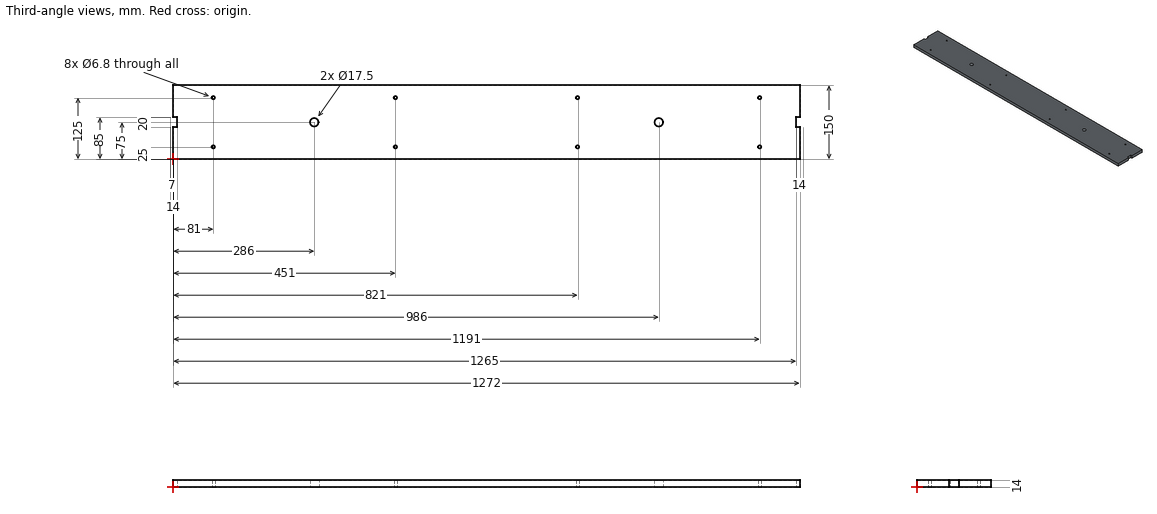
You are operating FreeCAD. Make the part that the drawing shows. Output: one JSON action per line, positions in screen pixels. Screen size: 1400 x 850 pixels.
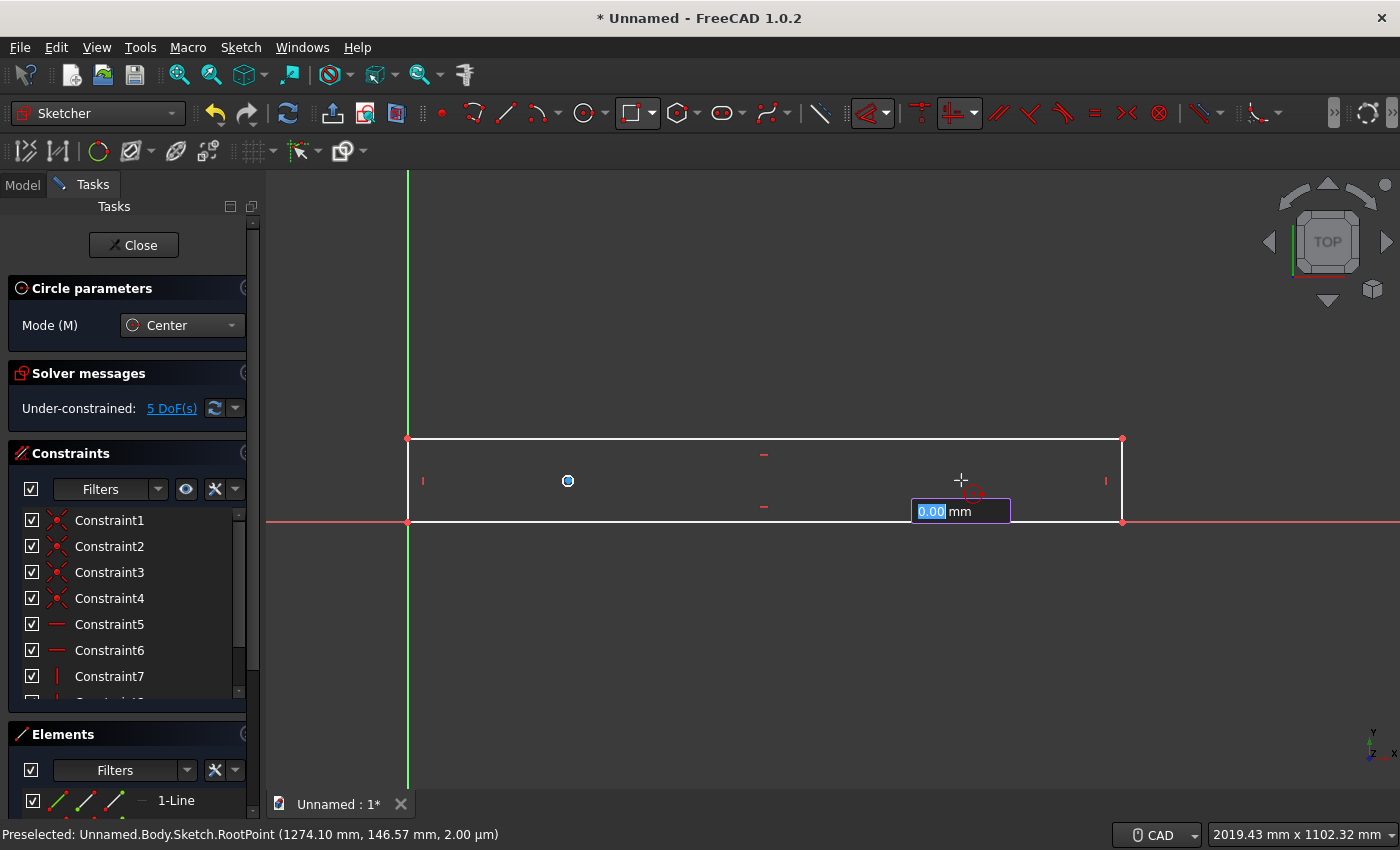
{"action": "scroll", "coordinate": [965, 477], "scroll_direction": "up", "scroll_amount": 6}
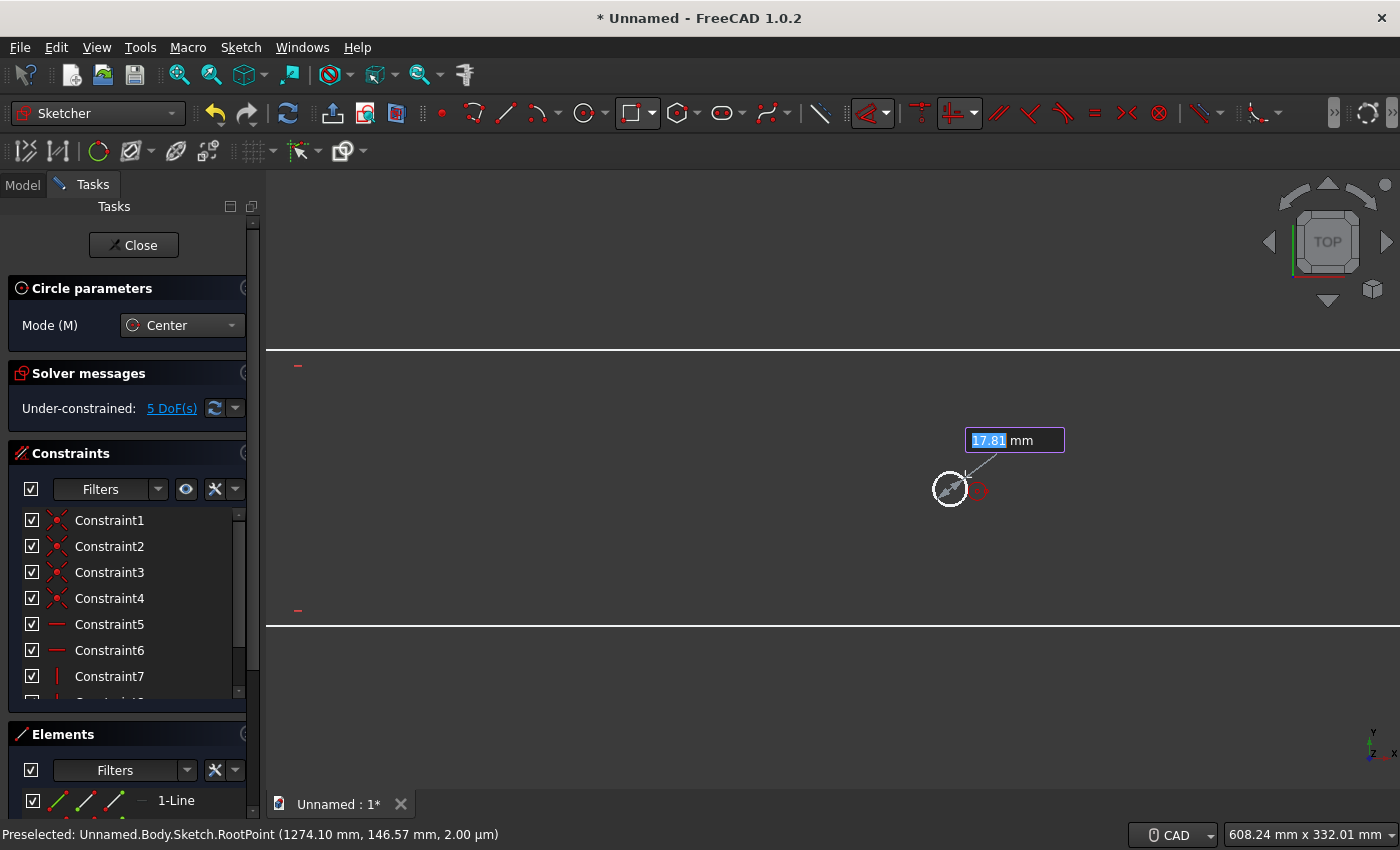
{"action": "left_click", "coordinate": [963, 475]}
{"action": "key", "text": "Escape"}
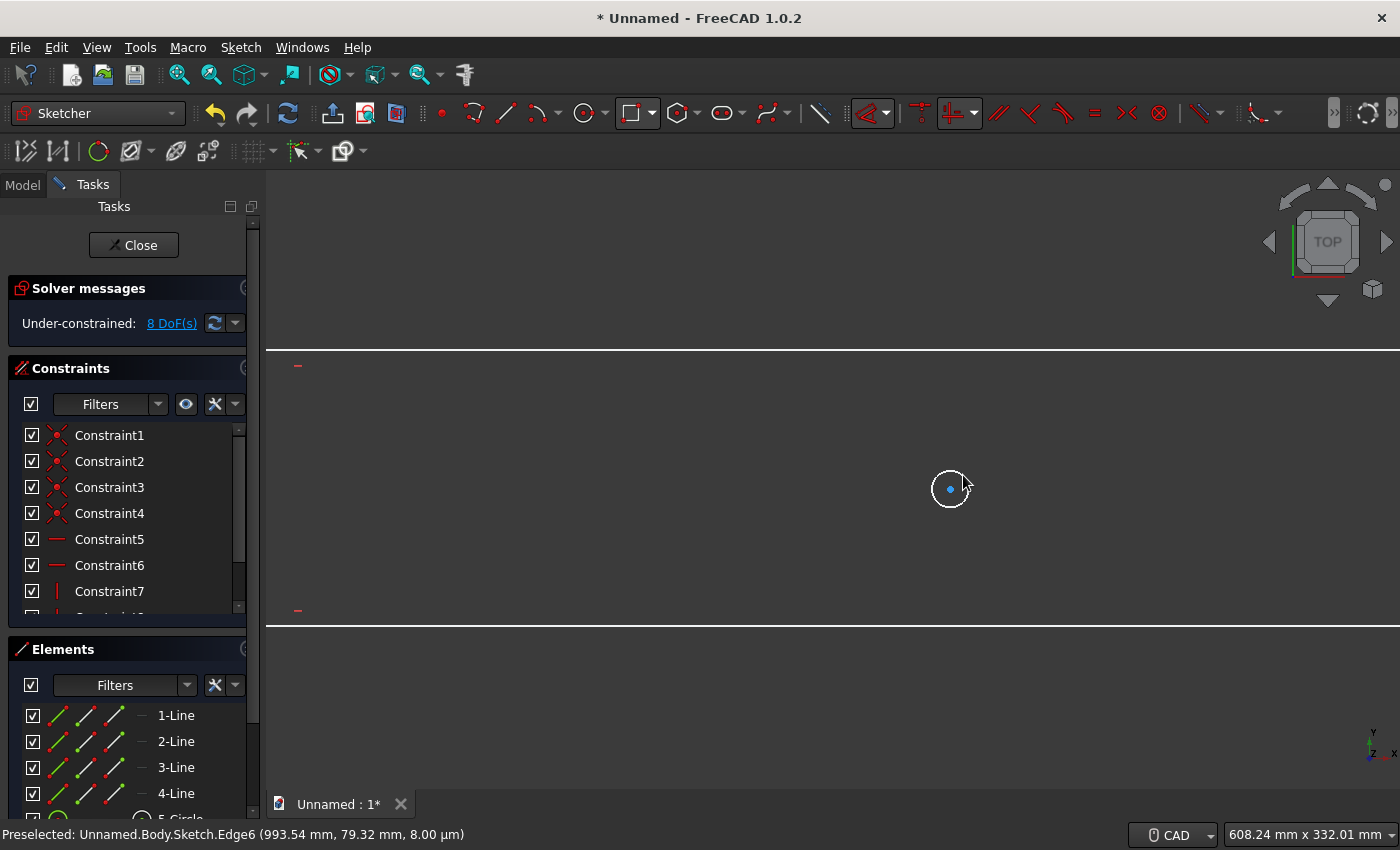
{"action": "scroll", "coordinate": [965, 477], "scroll_direction": "down", "scroll_amount": 6}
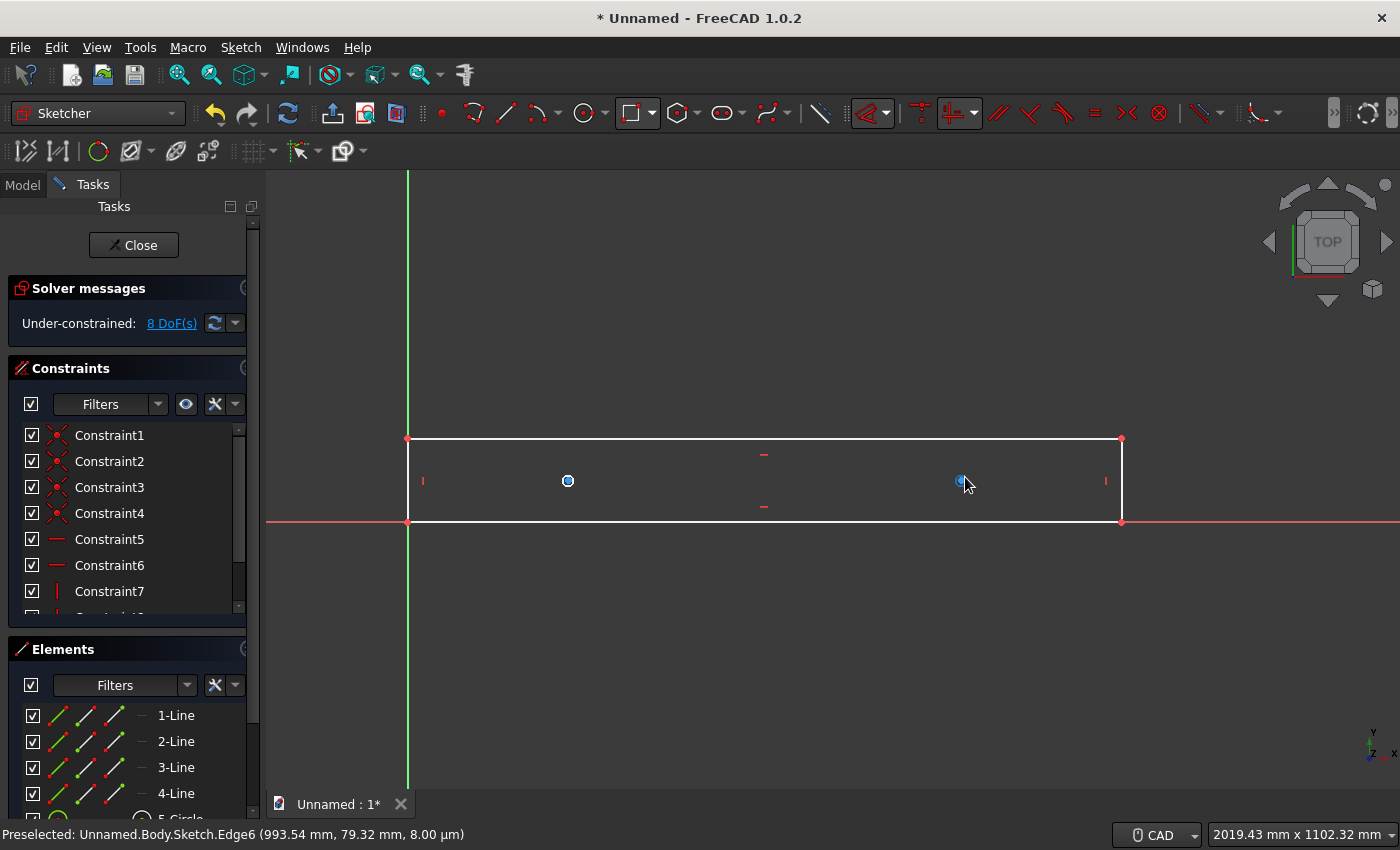
{"action": "scroll", "coordinate": [572, 477], "scroll_direction": "up", "scroll_amount": 5}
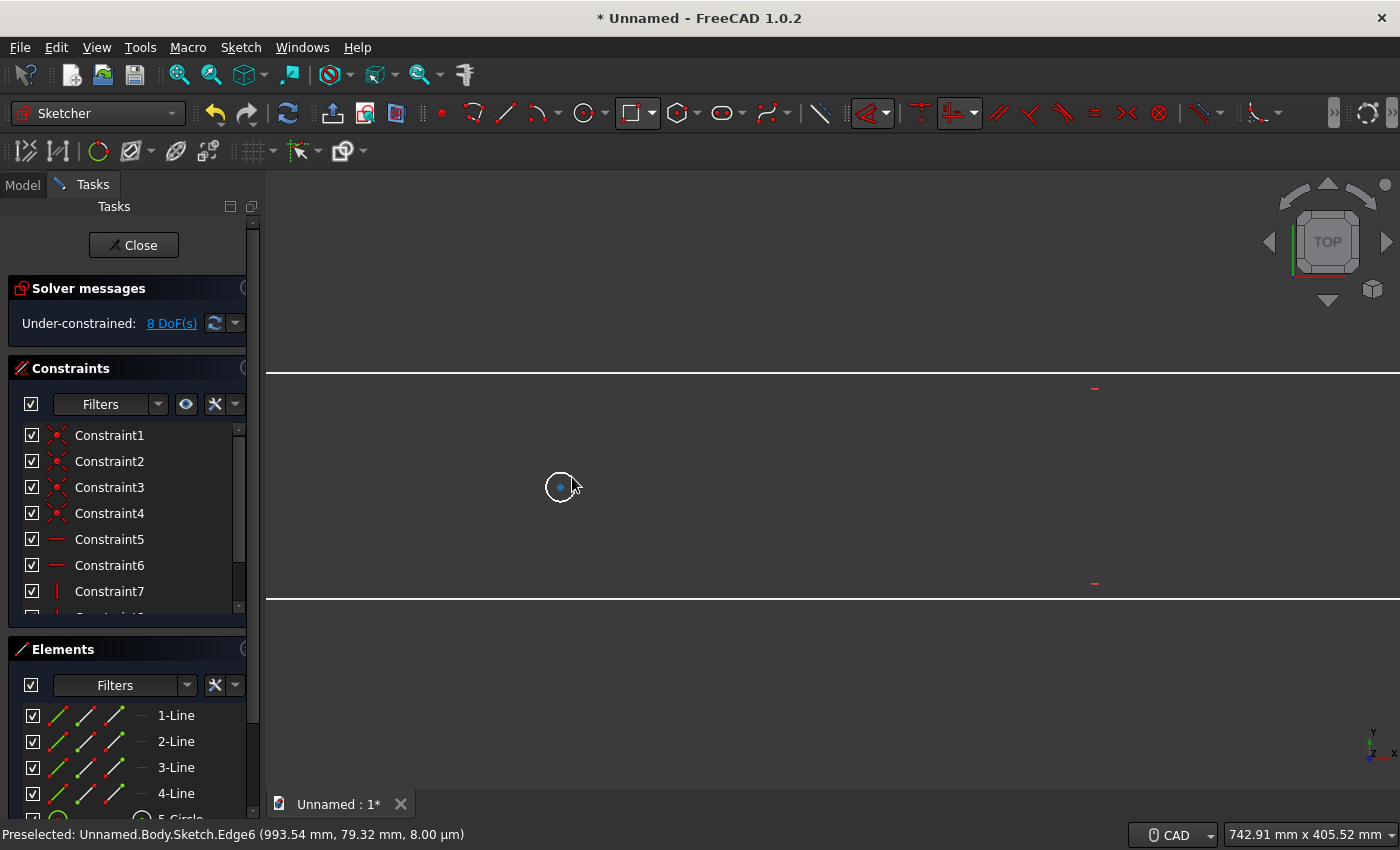
{"action": "left_click", "coordinate": [571, 477]}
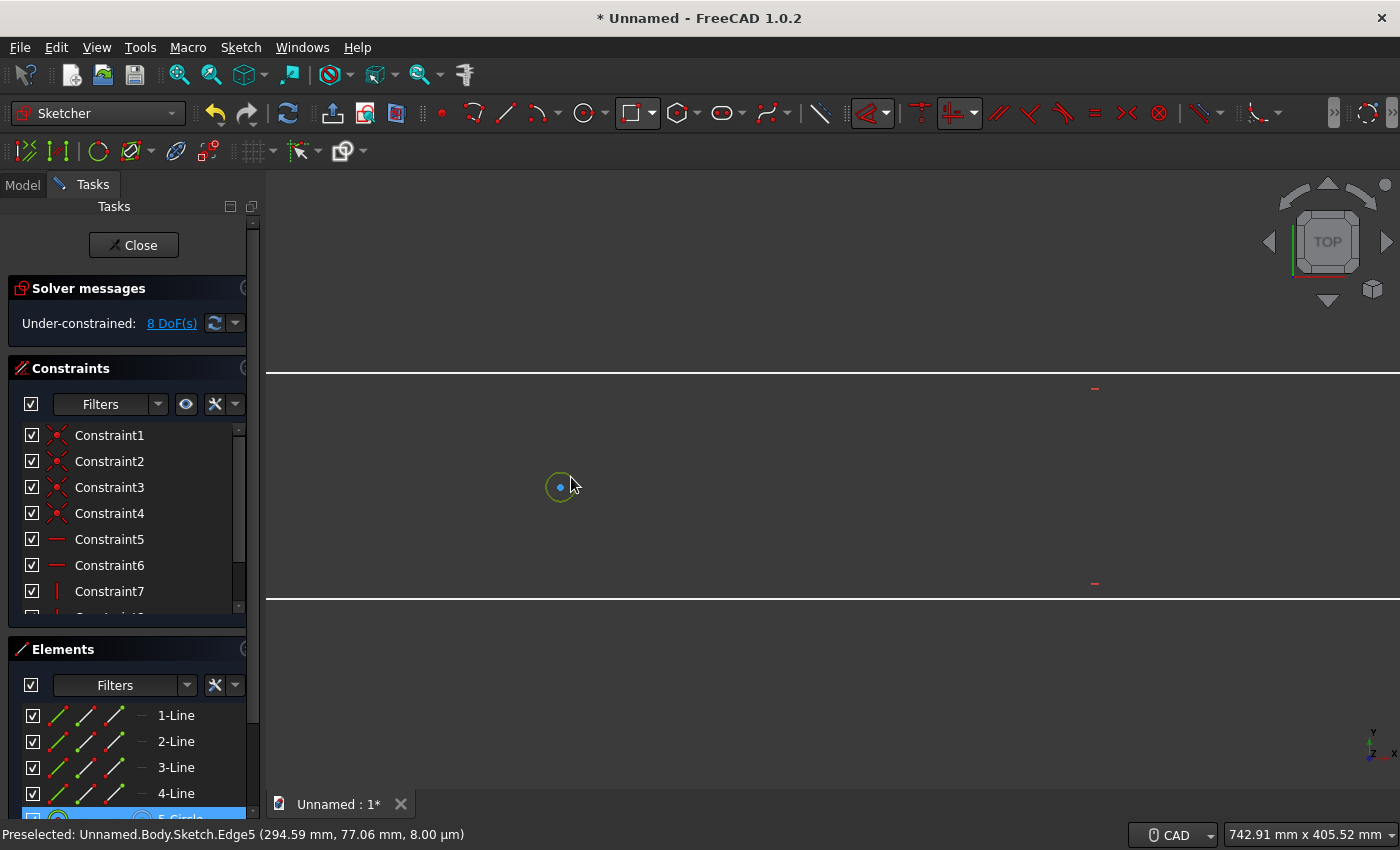
{"action": "scroll", "coordinate": [572, 476], "scroll_direction": "down", "scroll_amount": 5}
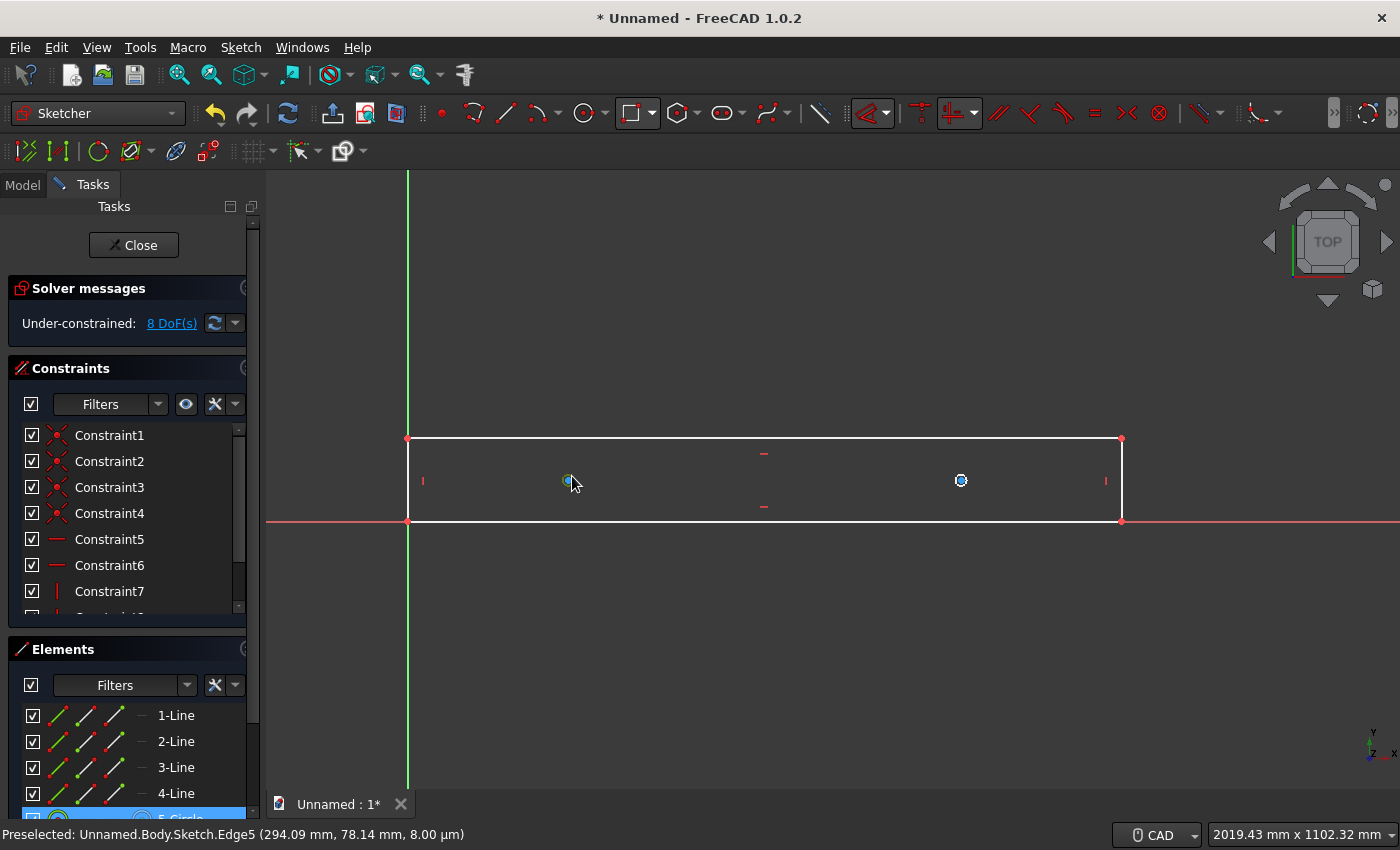
{"action": "scroll", "coordinate": [965, 476], "scroll_direction": "up", "scroll_amount": 5}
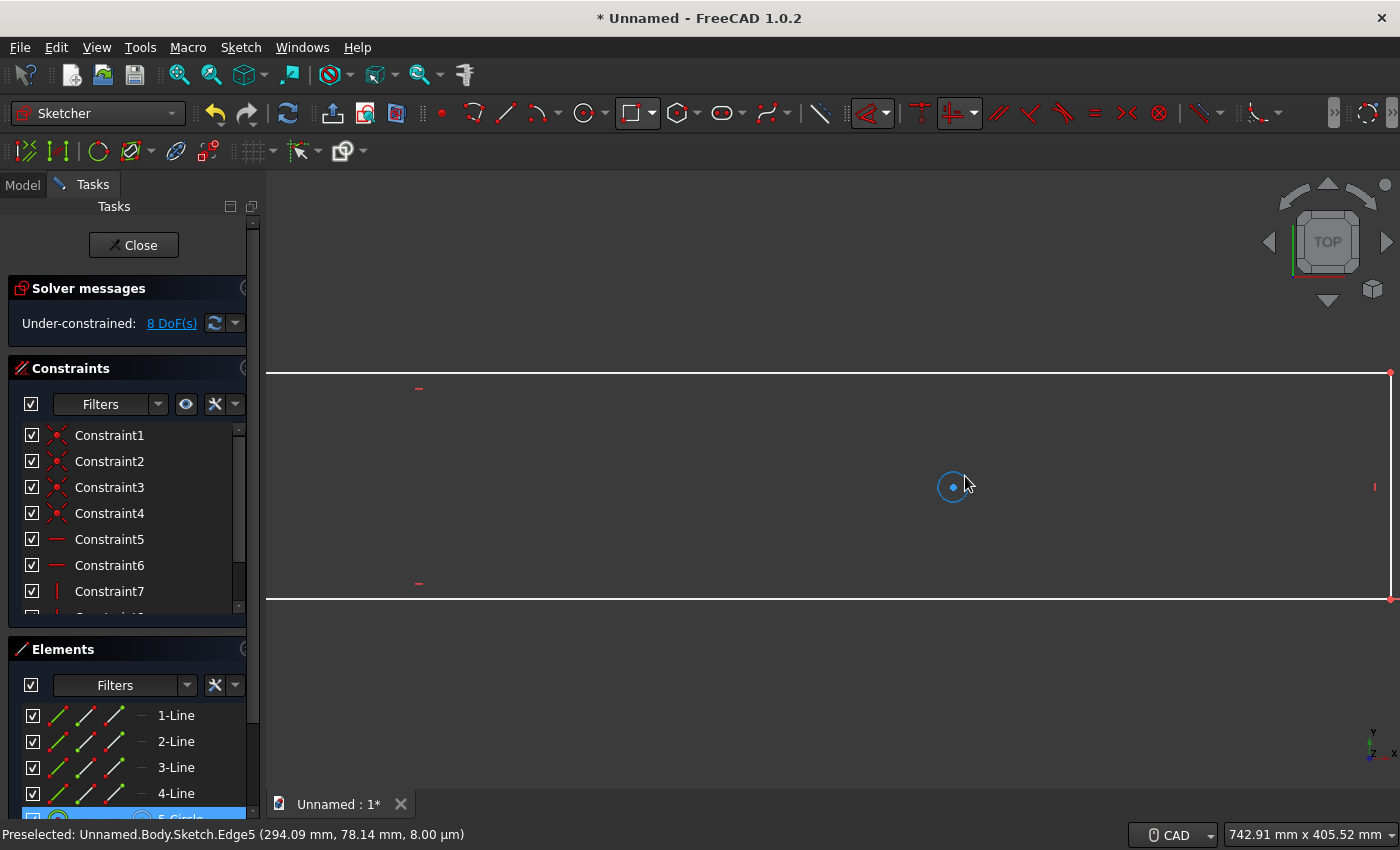
{"action": "left_click", "coordinate": [964, 476]}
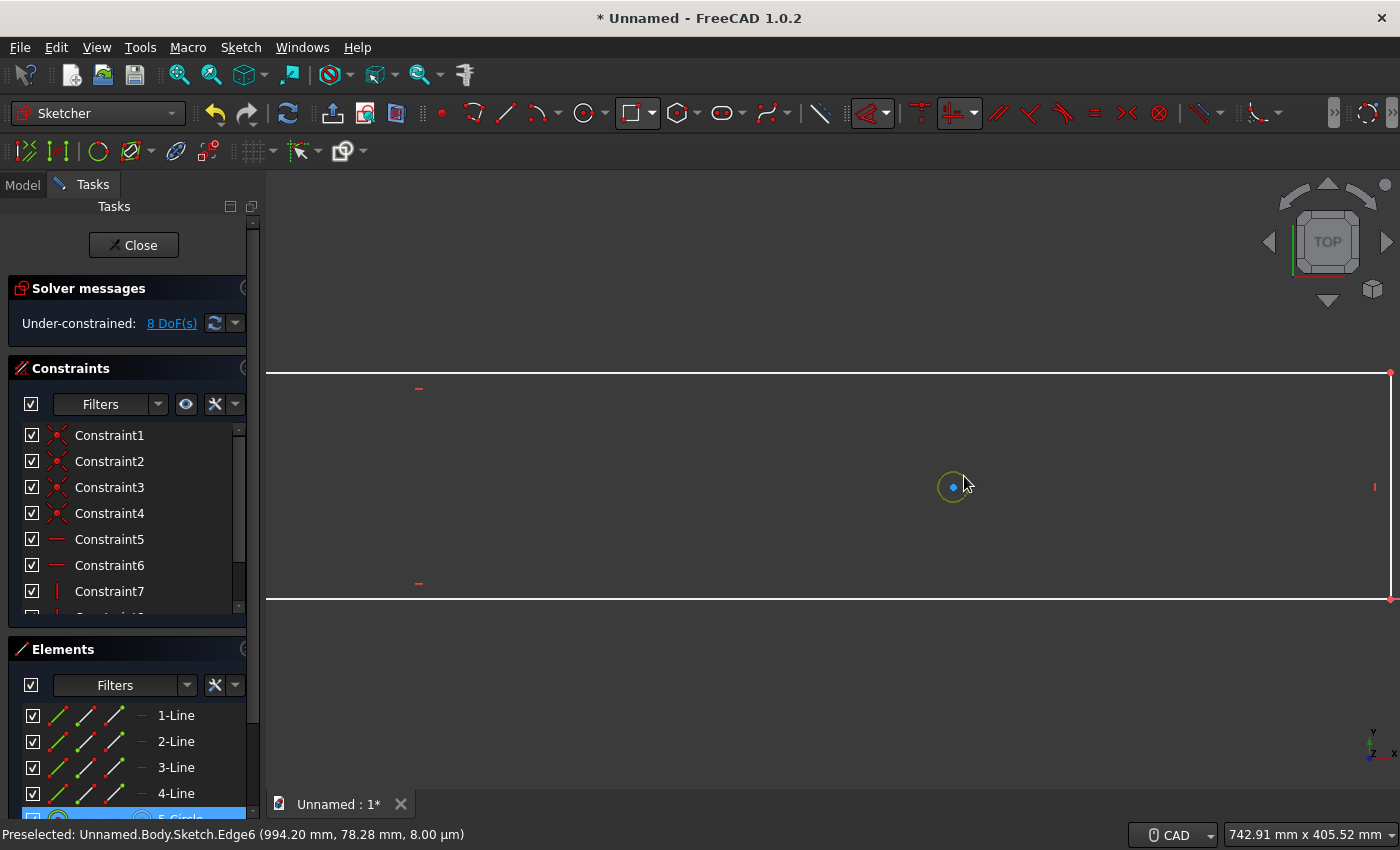
{"action": "left_click", "coordinate": [1096, 114]}